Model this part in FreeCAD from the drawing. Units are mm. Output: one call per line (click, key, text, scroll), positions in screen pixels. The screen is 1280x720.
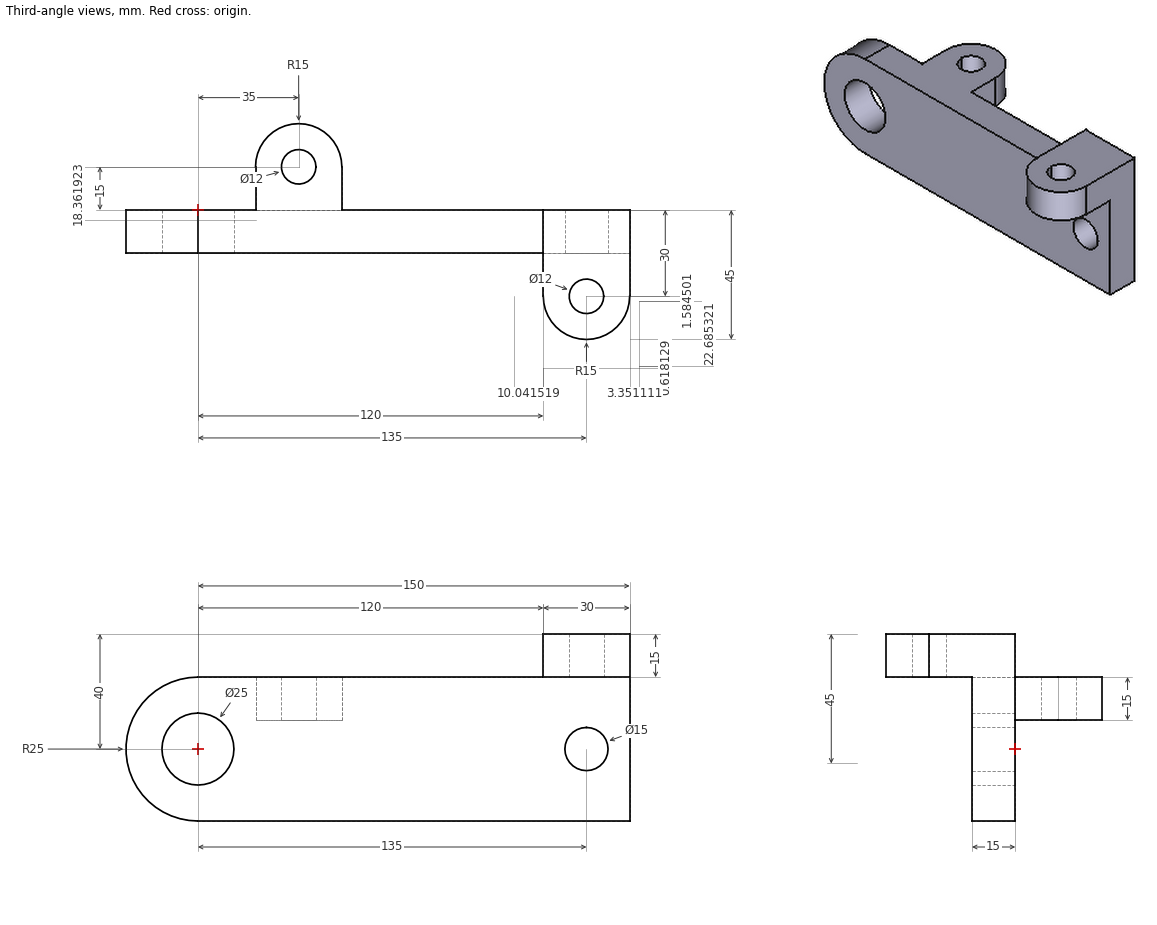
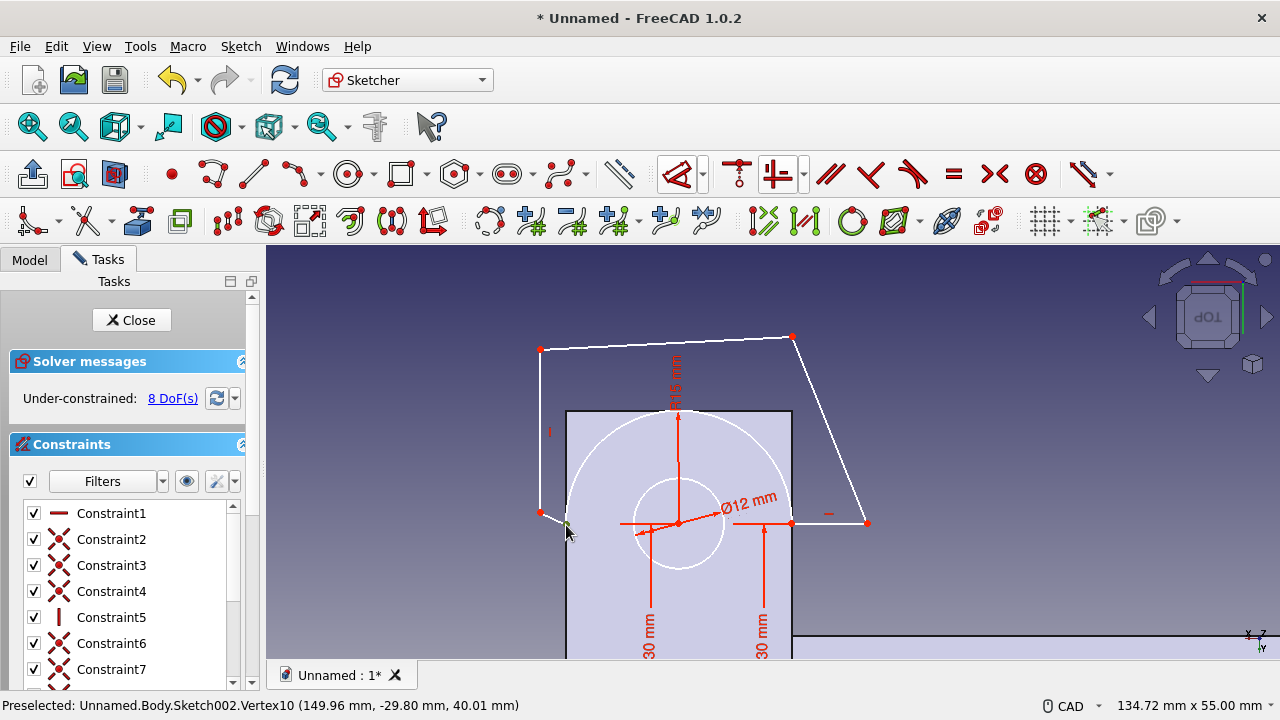
key(i)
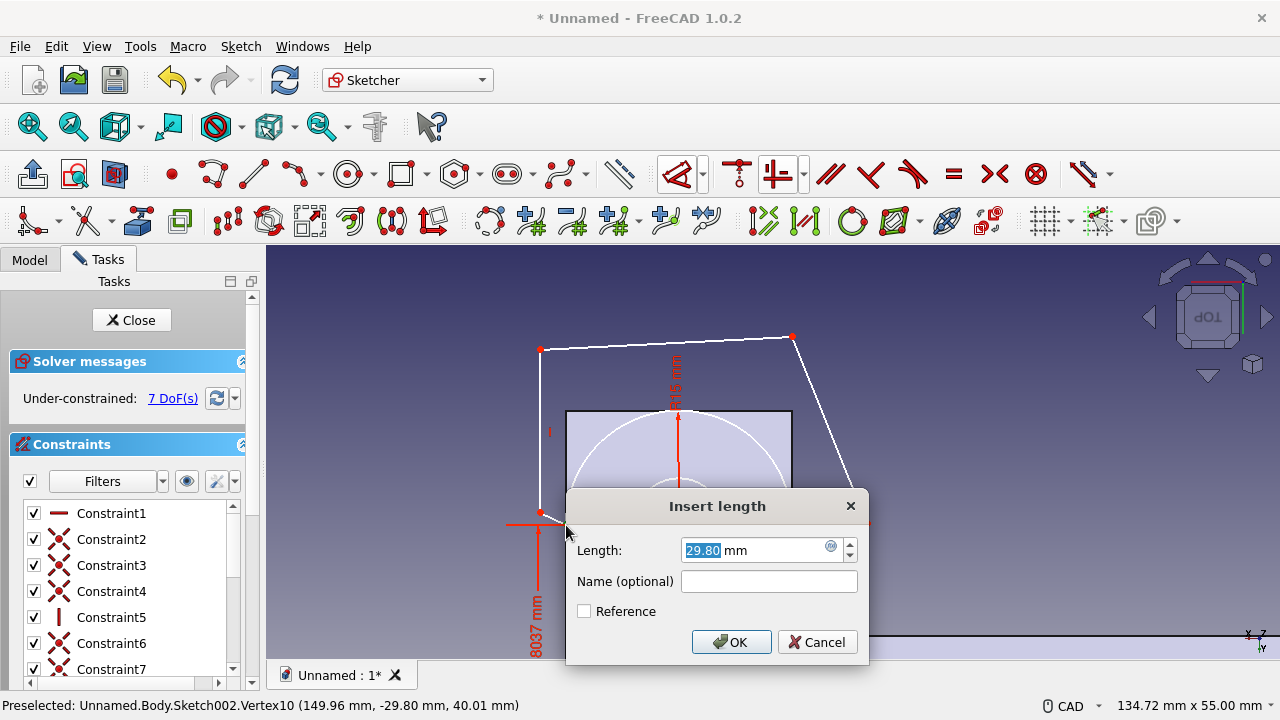
text(30)
key(Return)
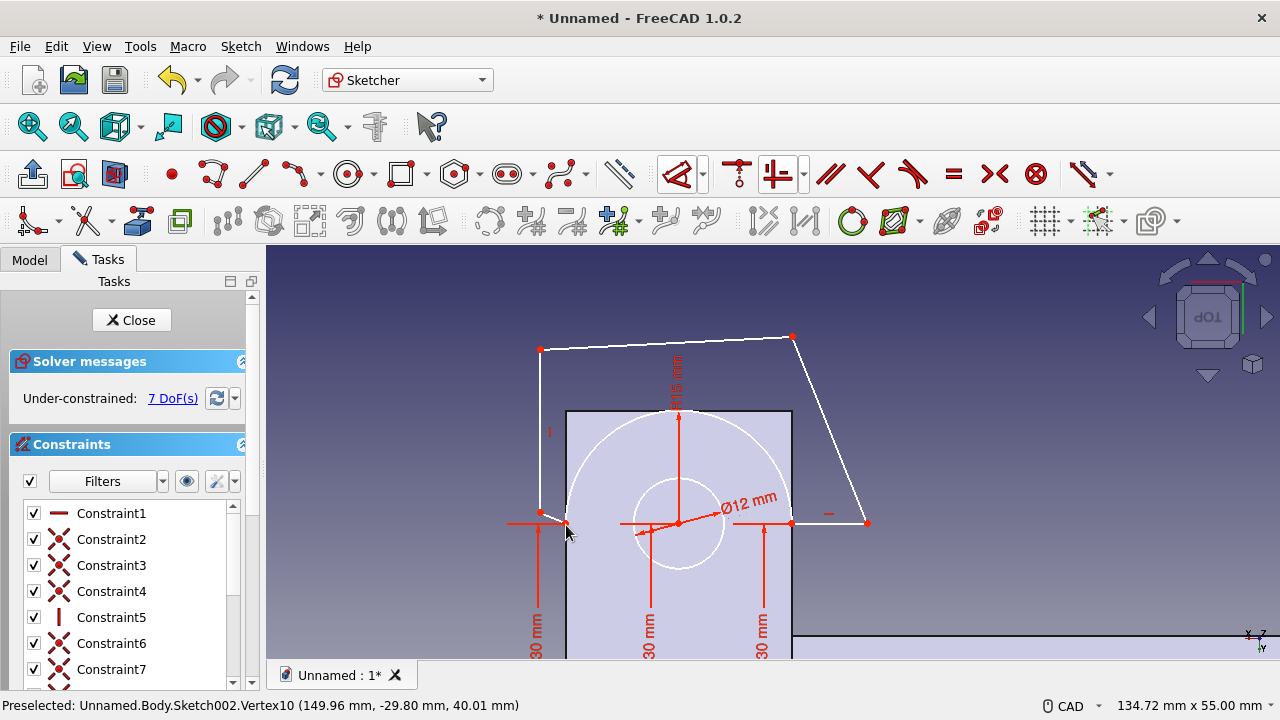
click(679, 524)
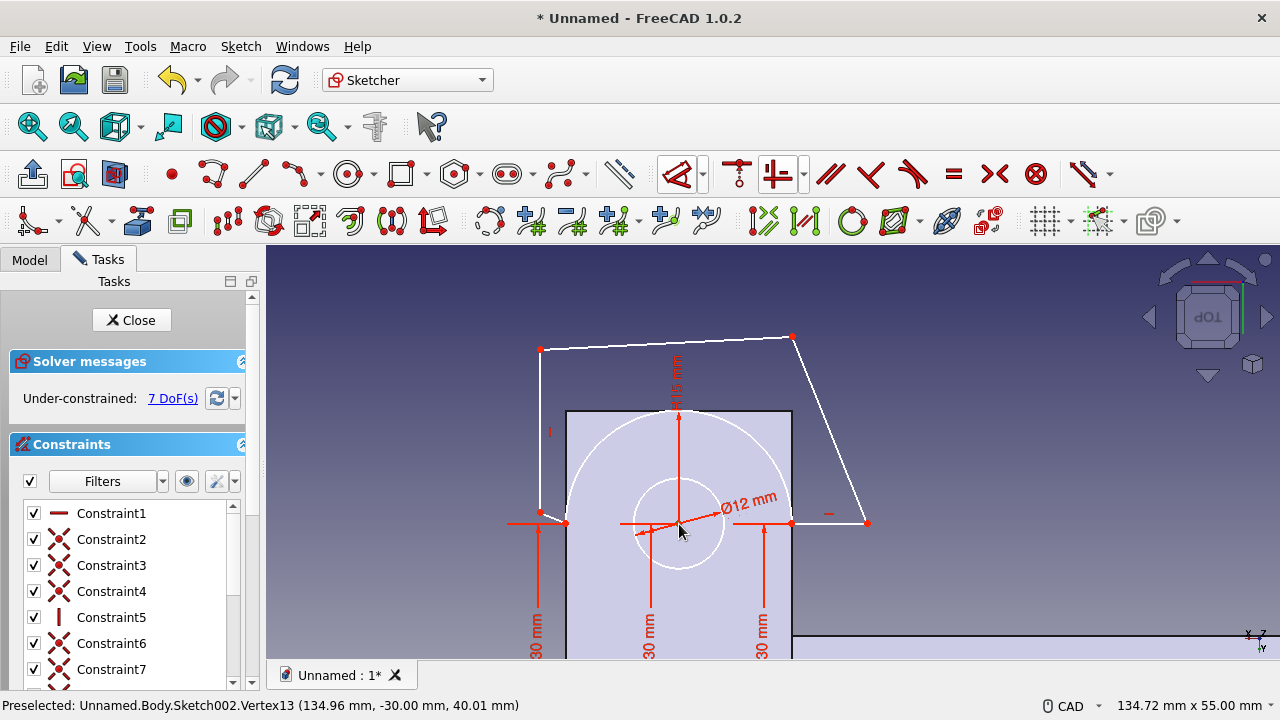
key(l)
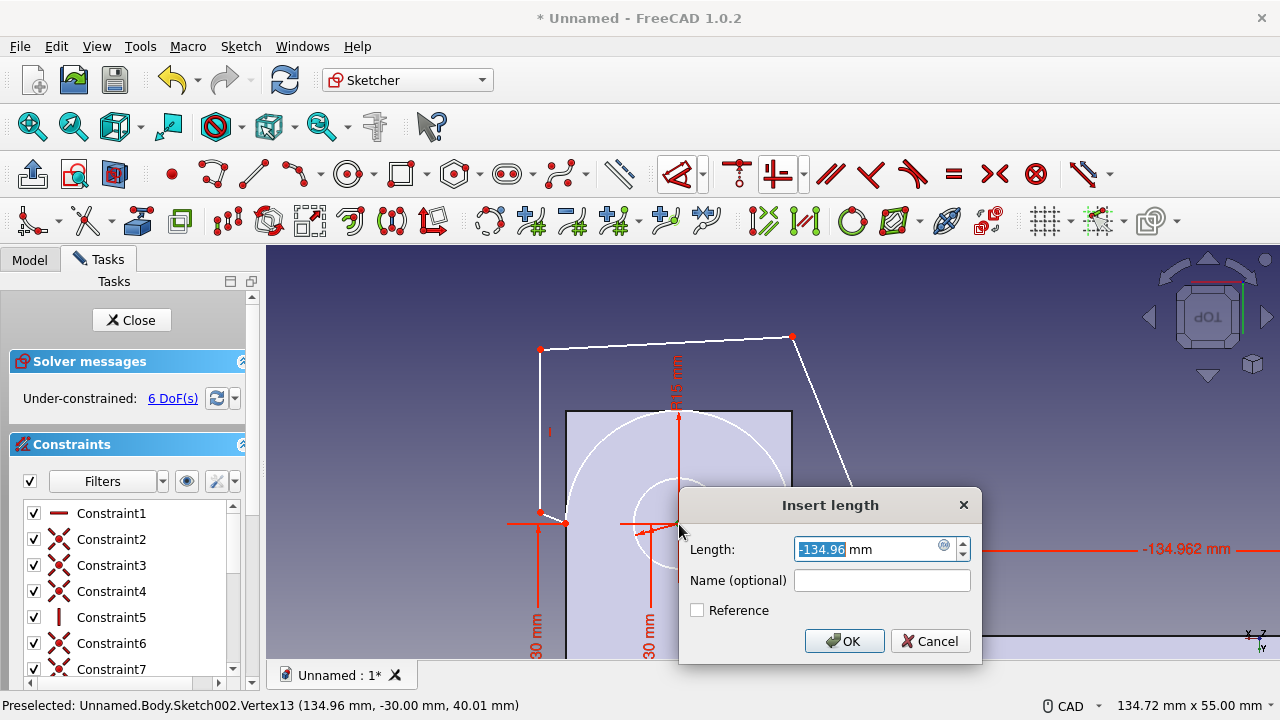
text(-135)
key(Return)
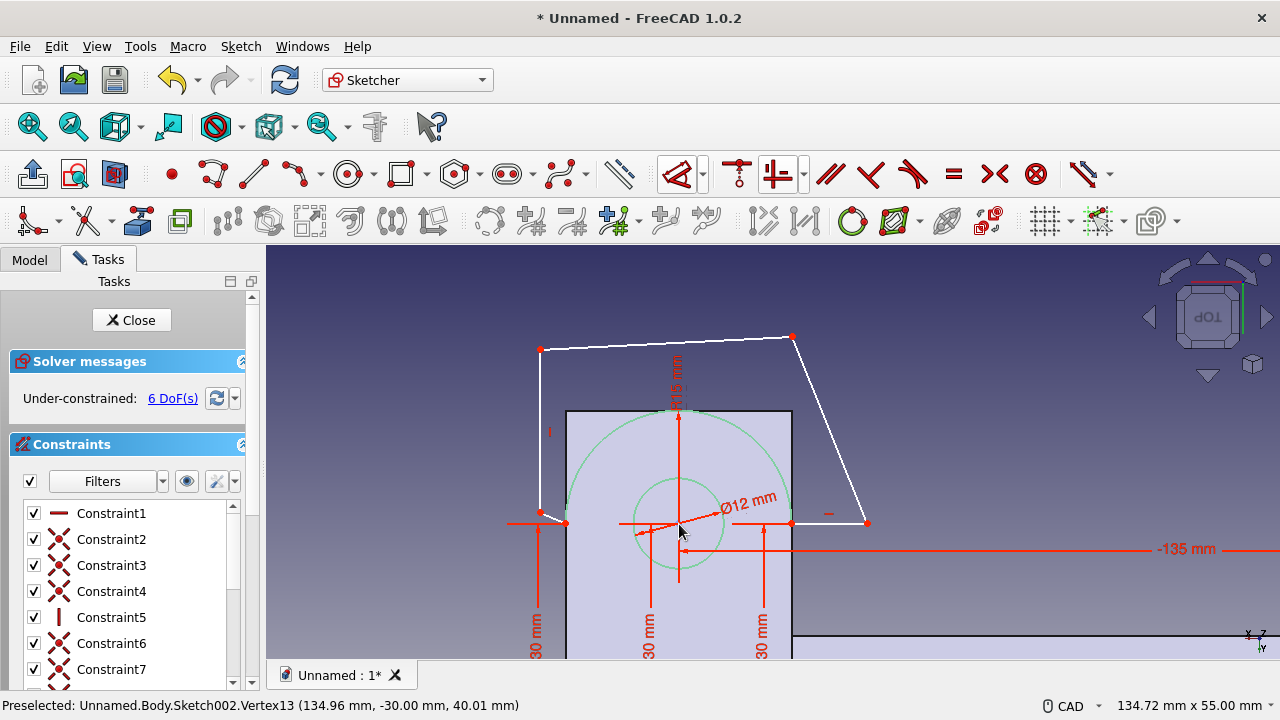
click(792, 337)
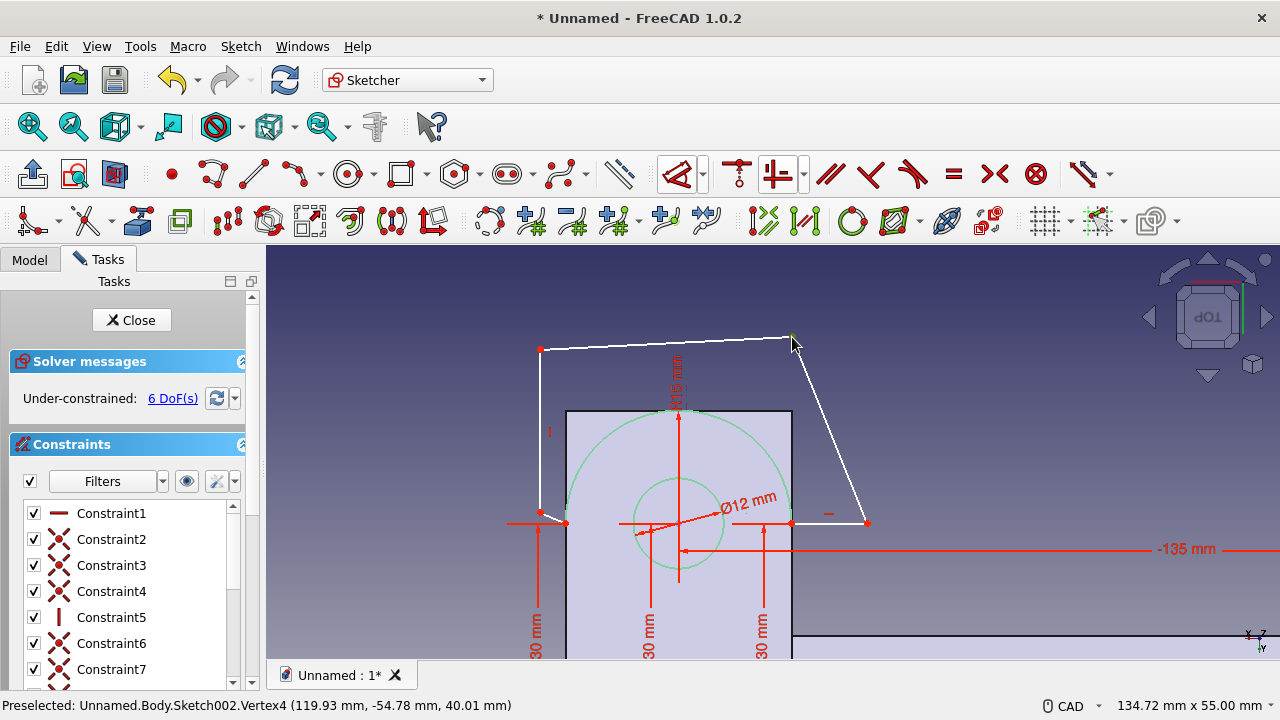
click(702, 174)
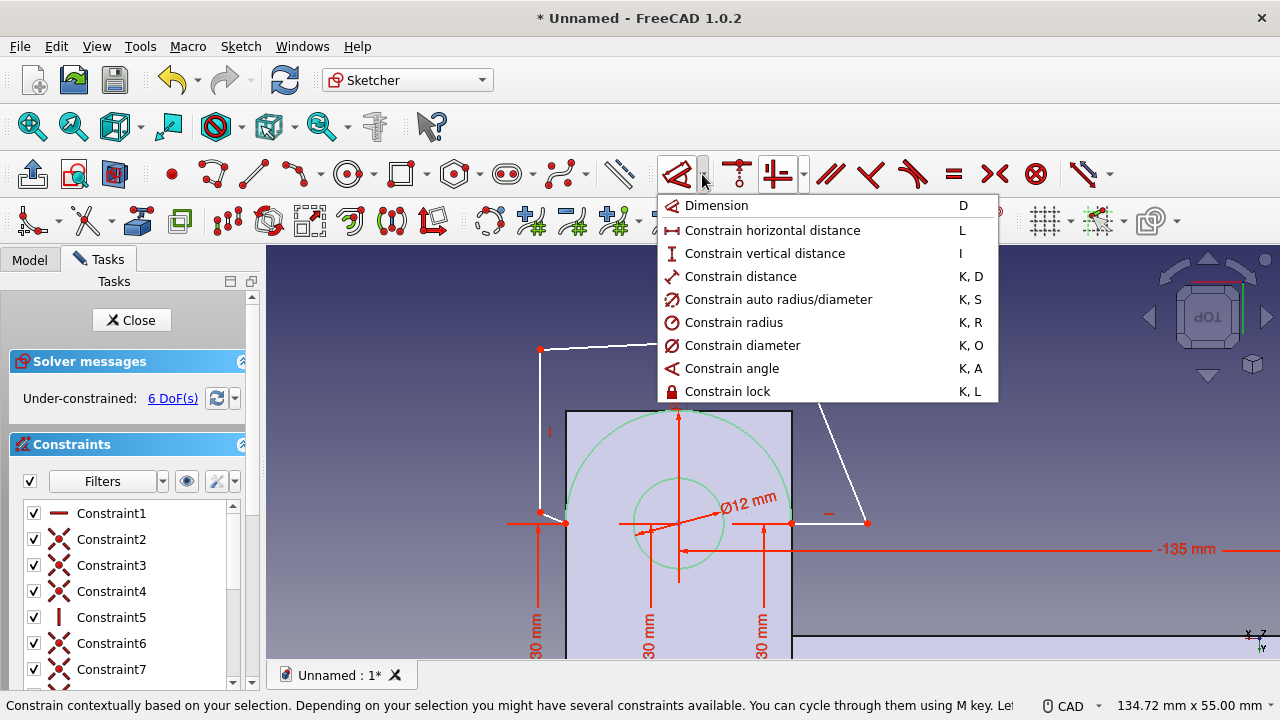
click(828, 230)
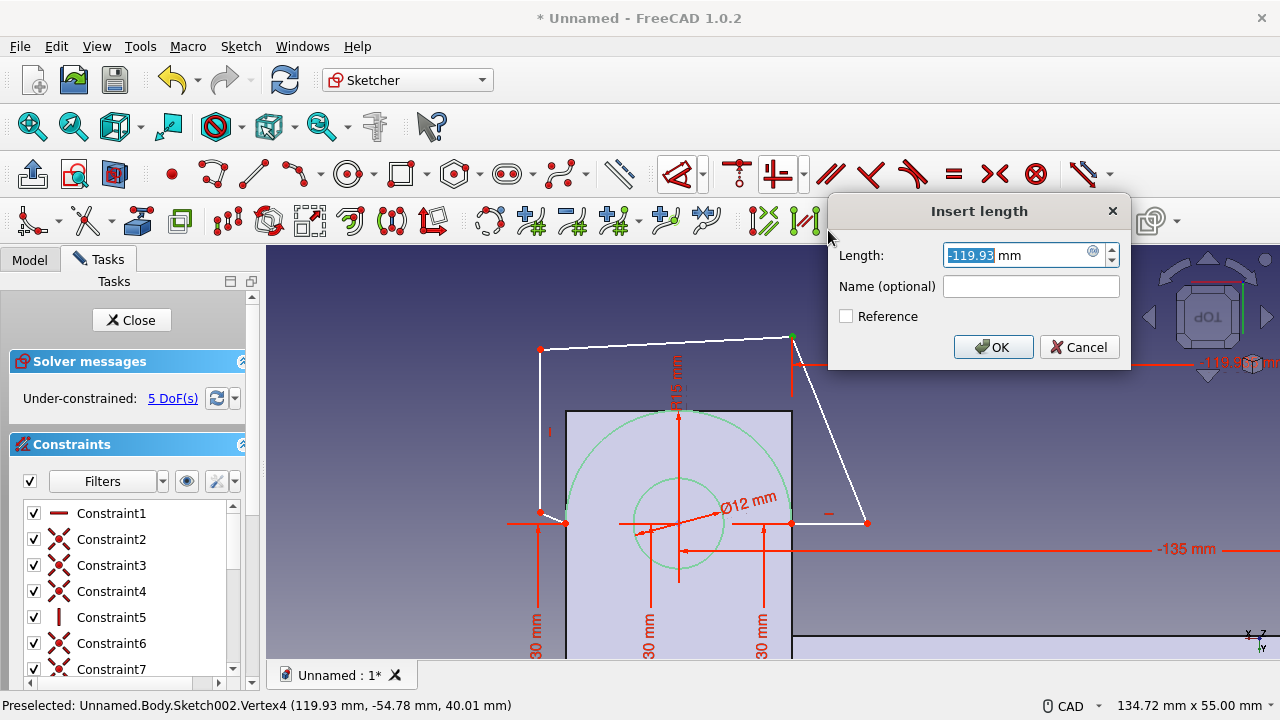
text(-120)
key(Return)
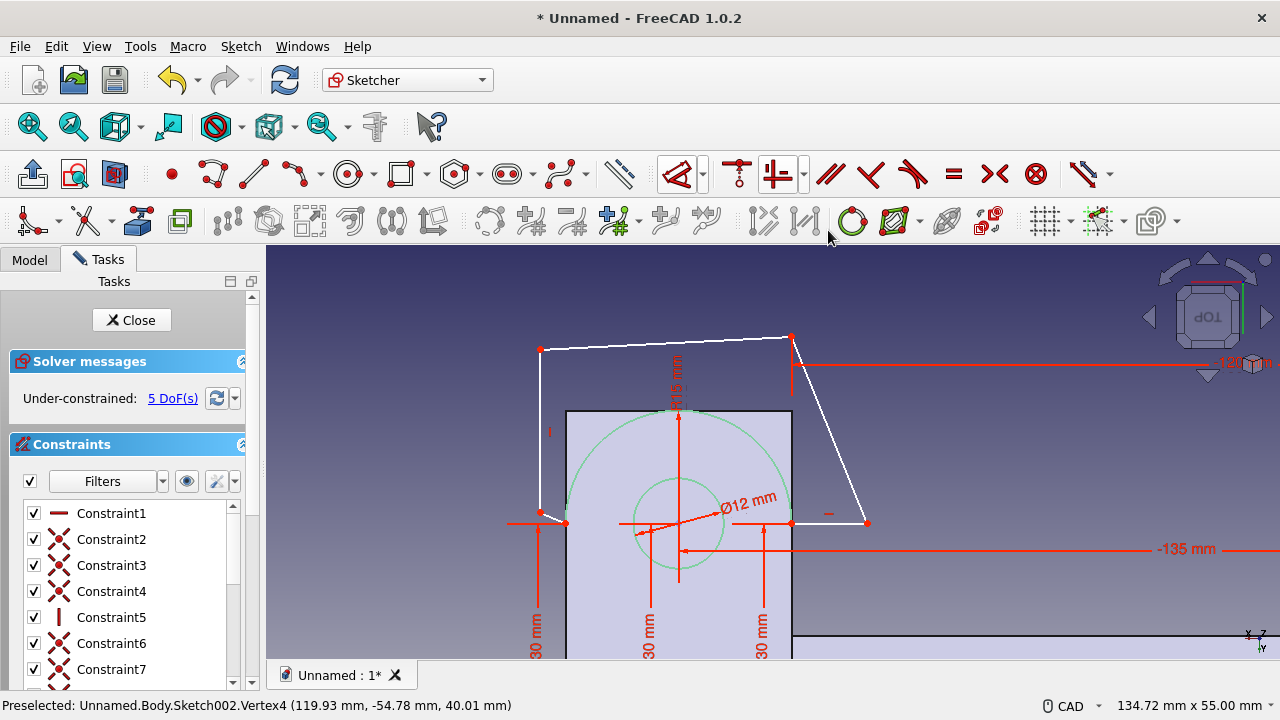
click(814, 524)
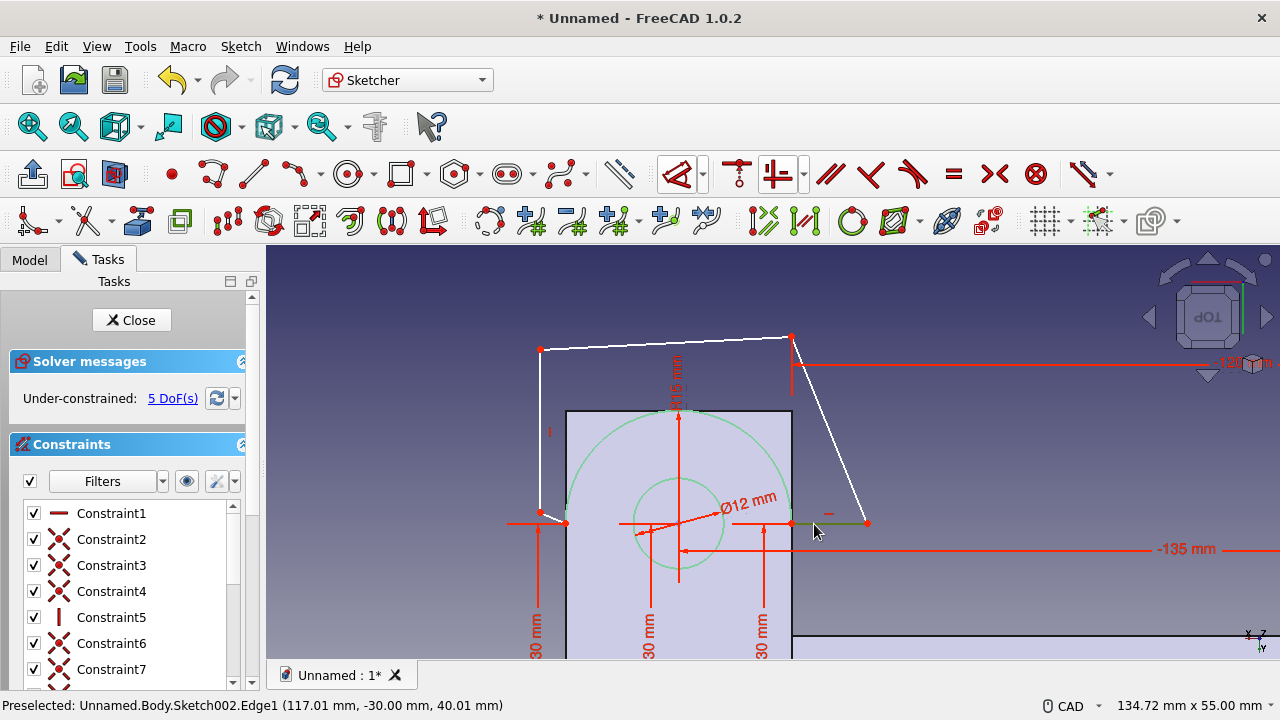
key(l)